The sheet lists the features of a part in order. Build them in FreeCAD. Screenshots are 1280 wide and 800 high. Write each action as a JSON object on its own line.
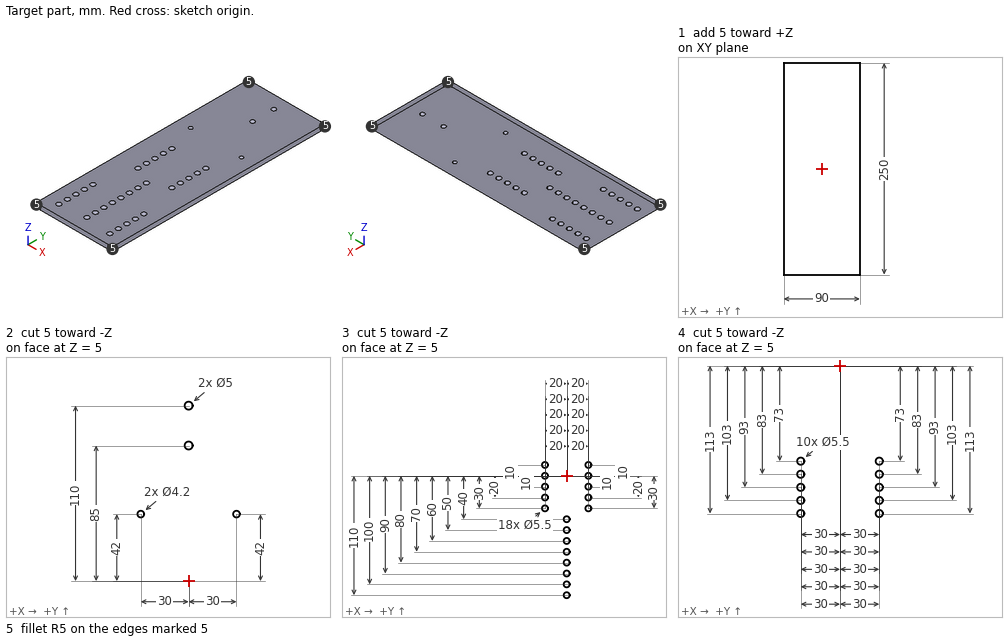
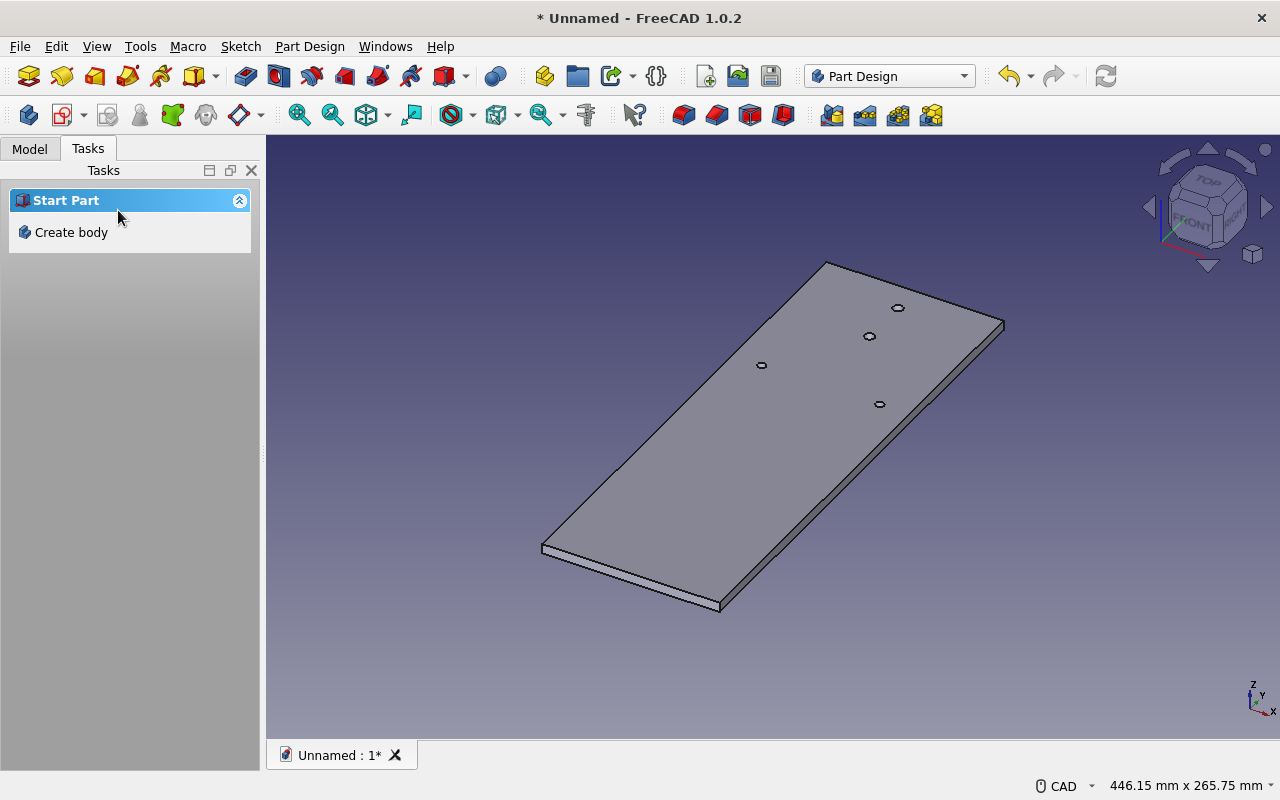
{"action": "left_click", "coordinate": [773, 431]}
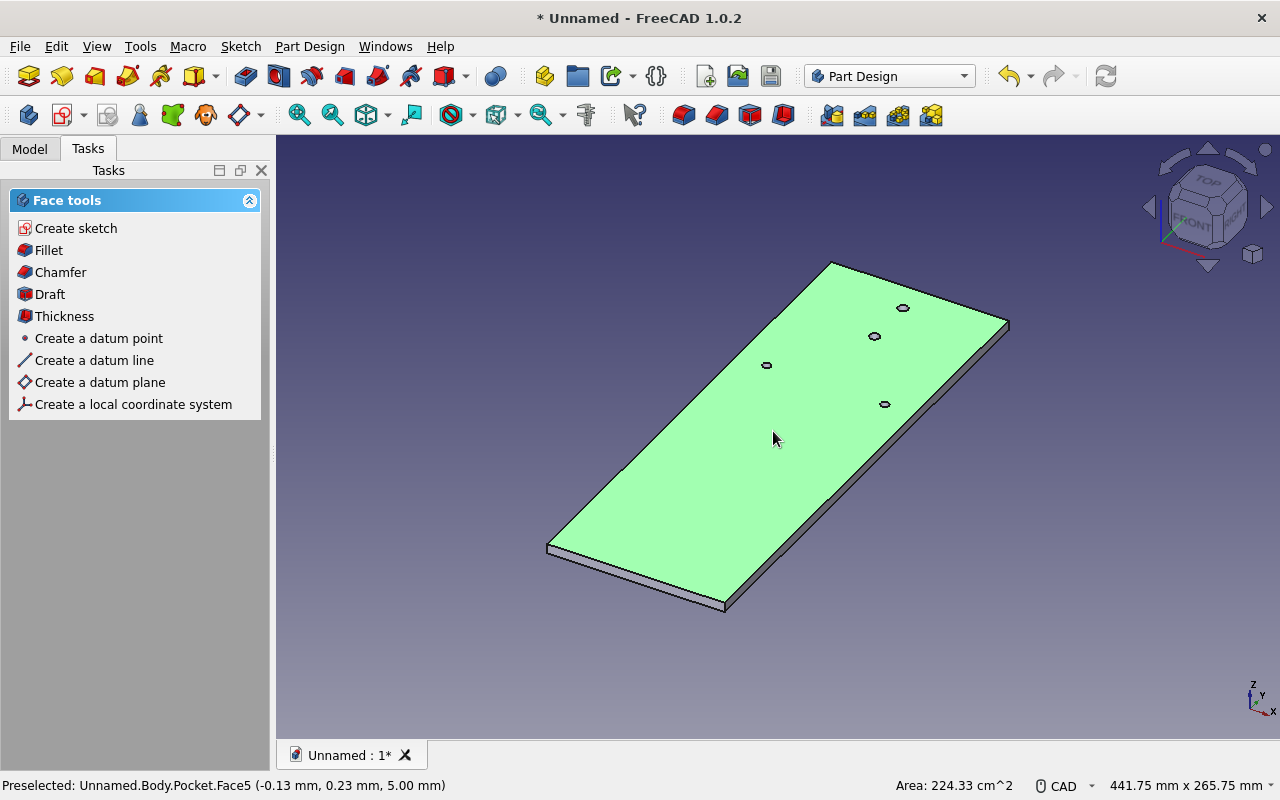
{"action": "left_click", "coordinate": [62, 116]}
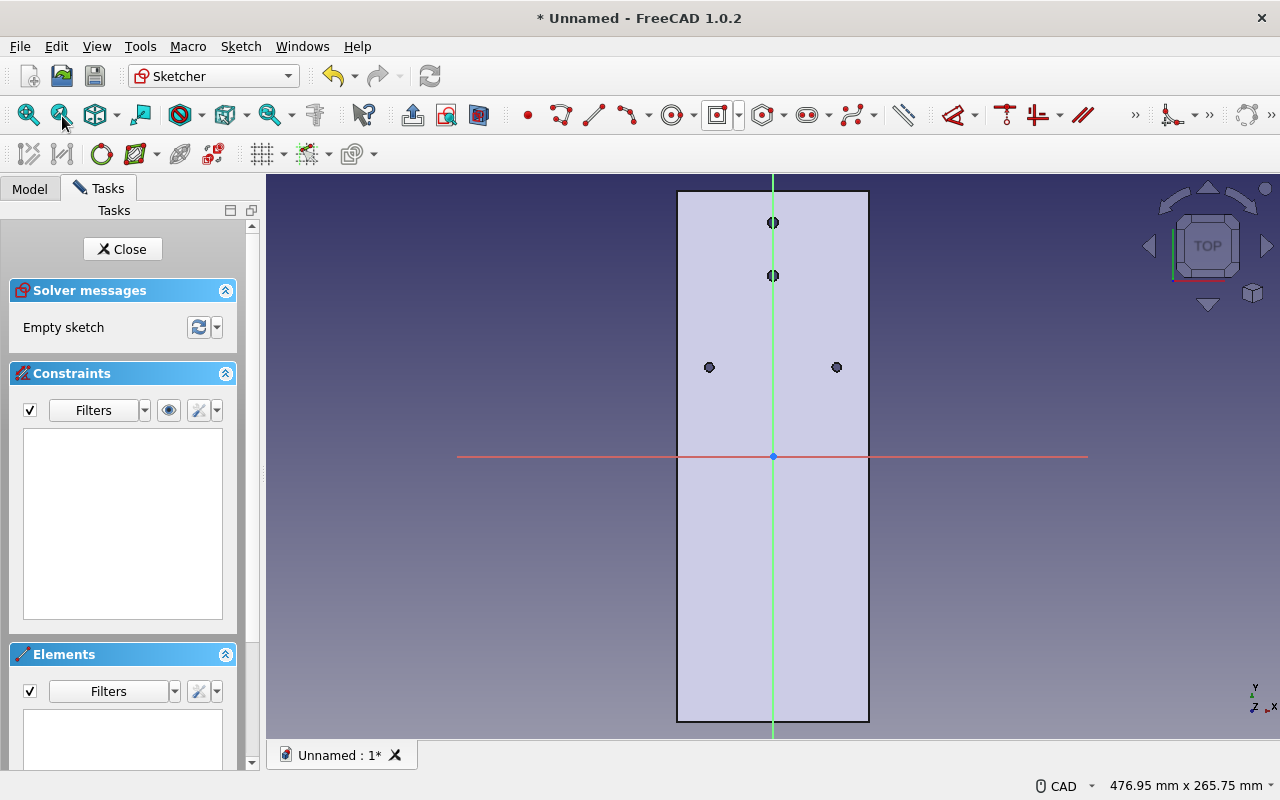
{"action": "scroll", "coordinate": [395, 202], "scroll_direction": "down", "scroll_amount": 1}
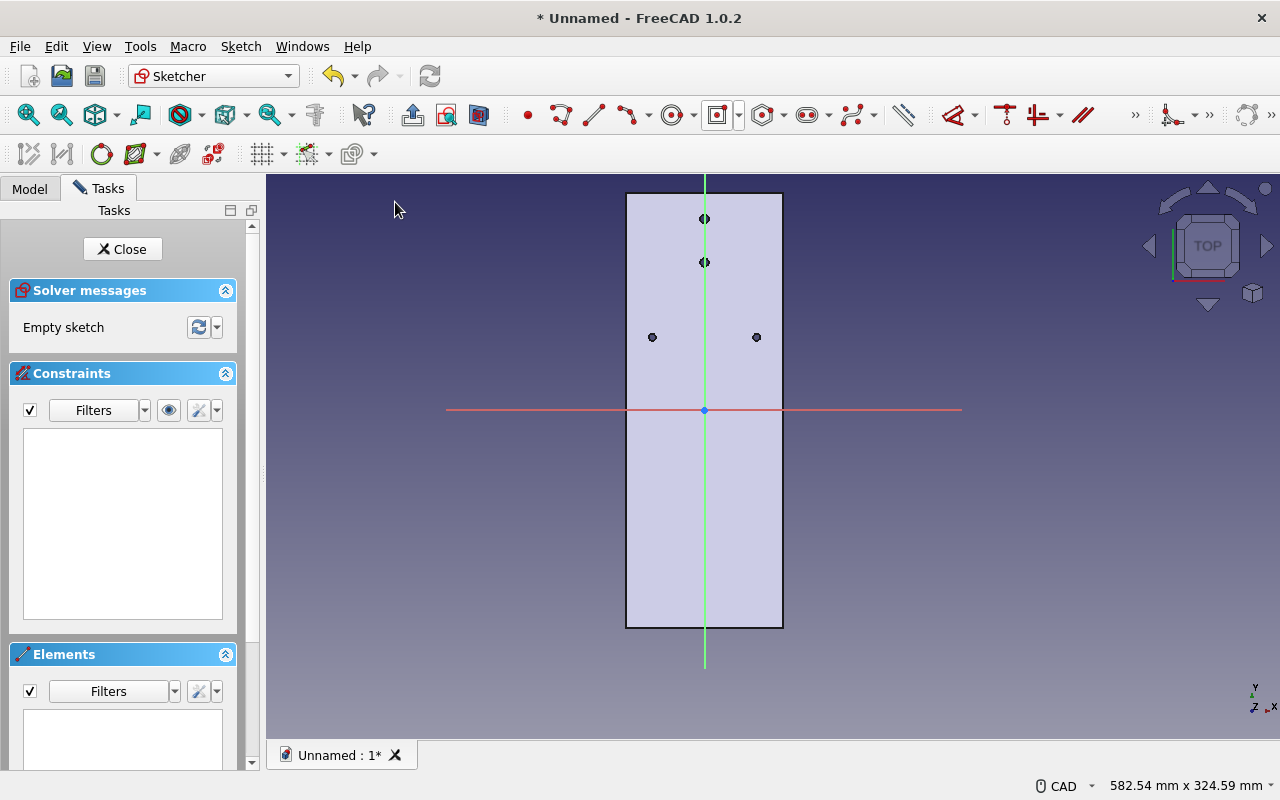
{"action": "scroll", "coordinate": [705, 581], "scroll_direction": "up", "scroll_amount": 2}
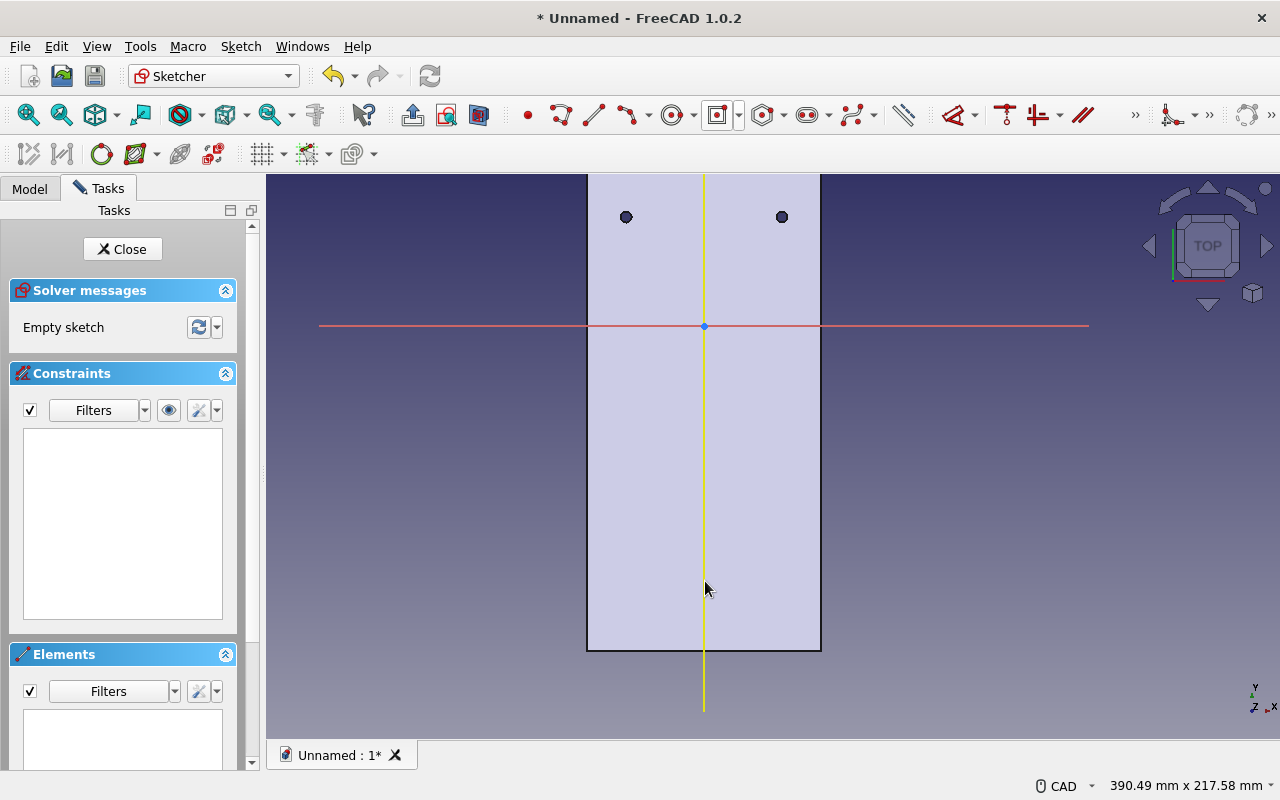
{"action": "key", "text": "g c"}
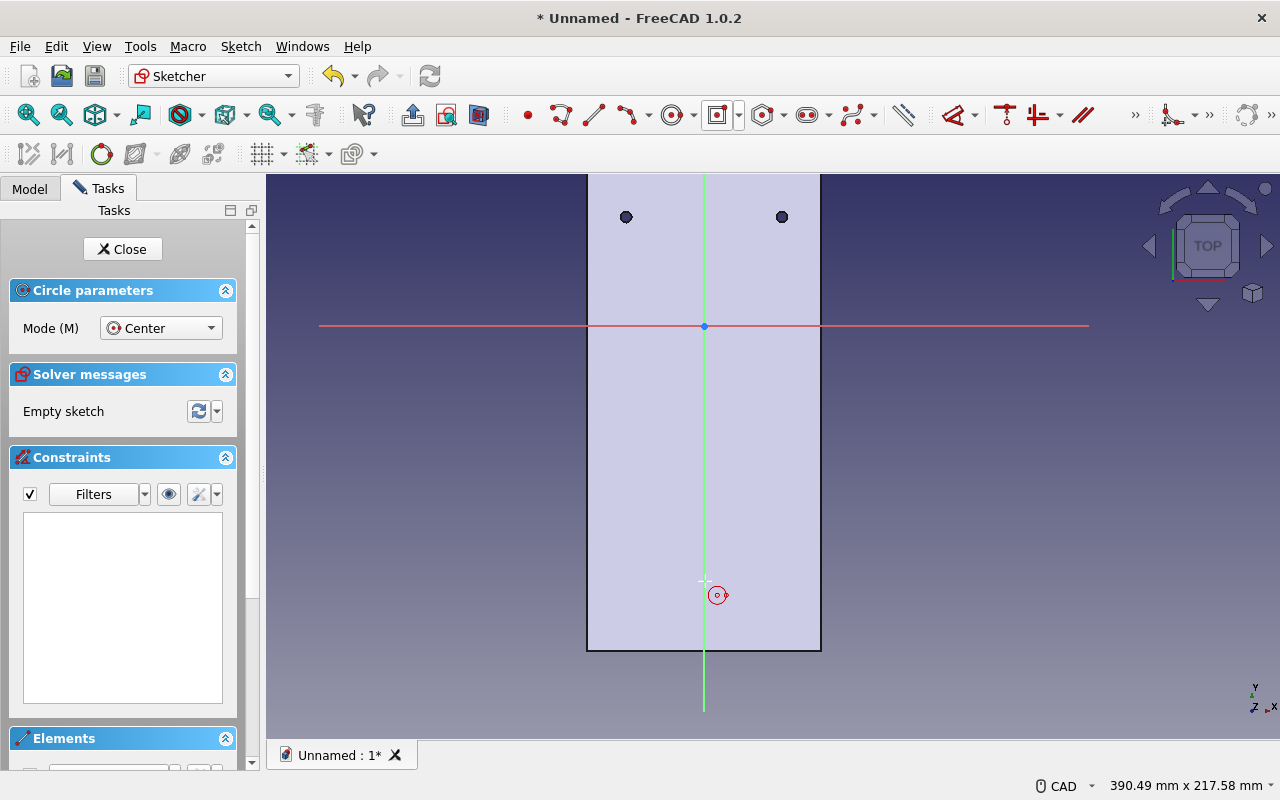
{"action": "scroll", "coordinate": [652, 404], "scroll_direction": "up", "scroll_amount": 6}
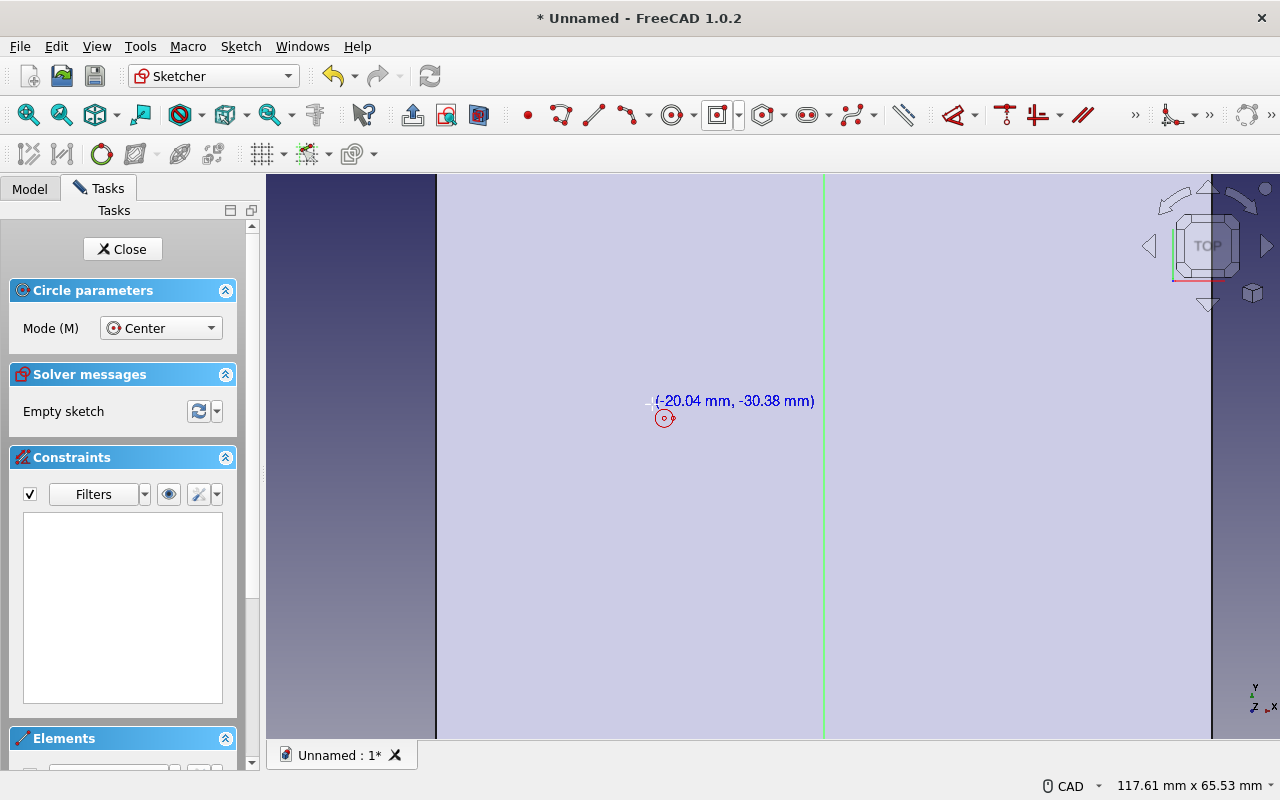
{"action": "left_click", "coordinate": [651, 403]}
{"action": "mouse_move", "coordinate": [668, 386]}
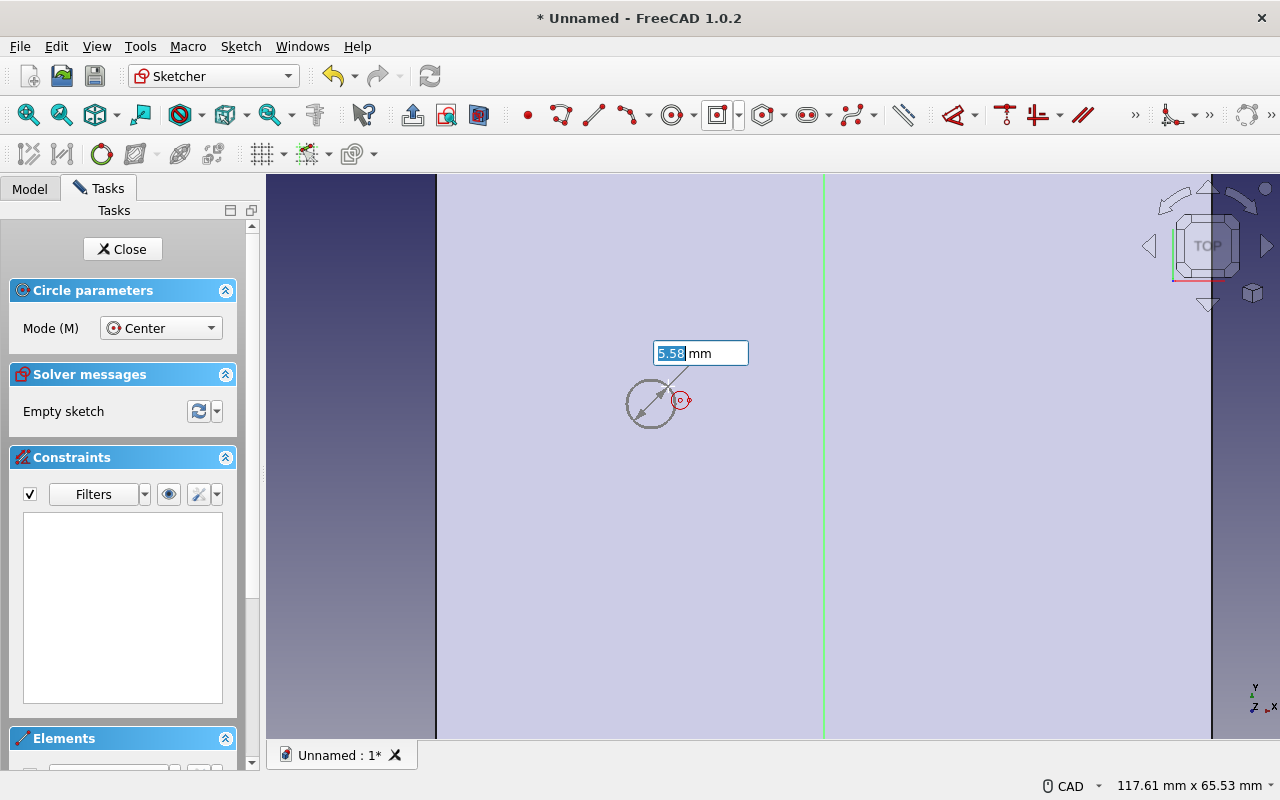
{"action": "type", "text": "5.5"}
{"action": "key", "text": "Return"}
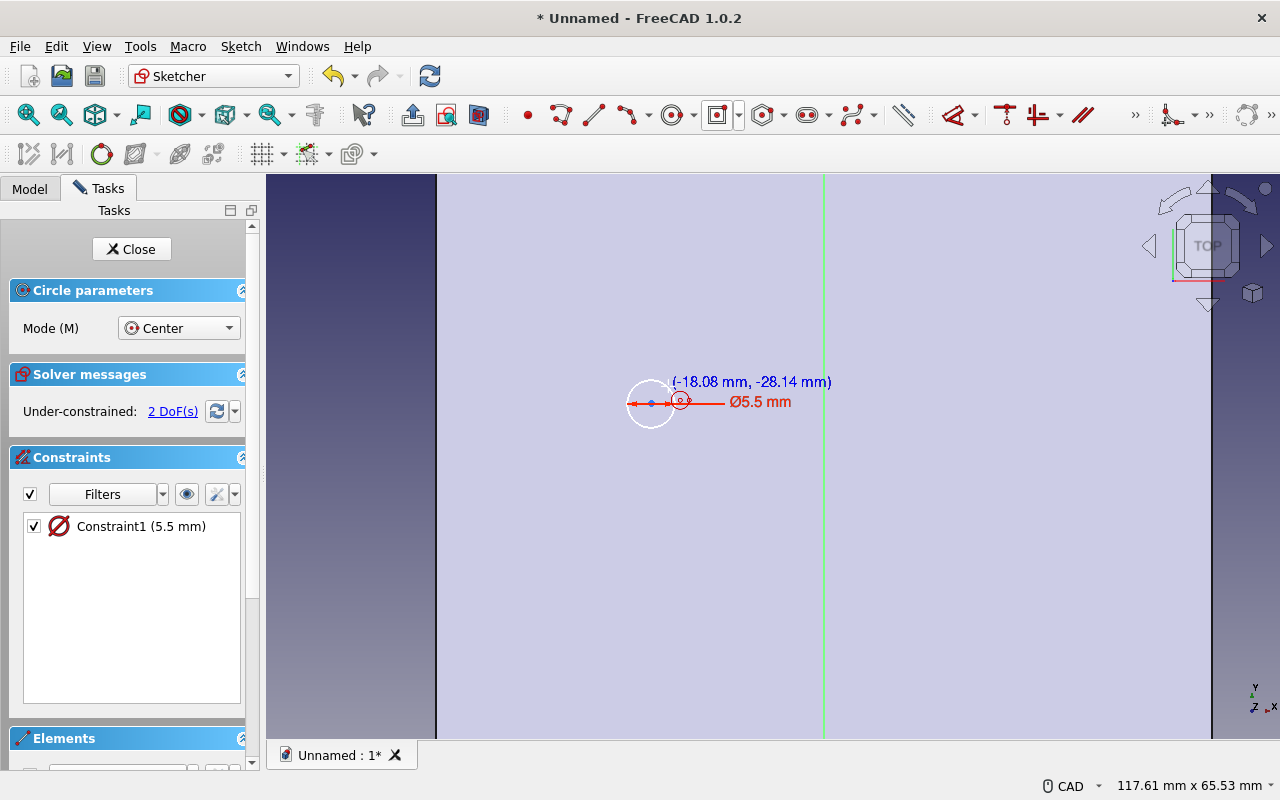
{"action": "left_click", "coordinate": [996, 403]}
{"action": "mouse_move", "coordinate": [1013, 386]}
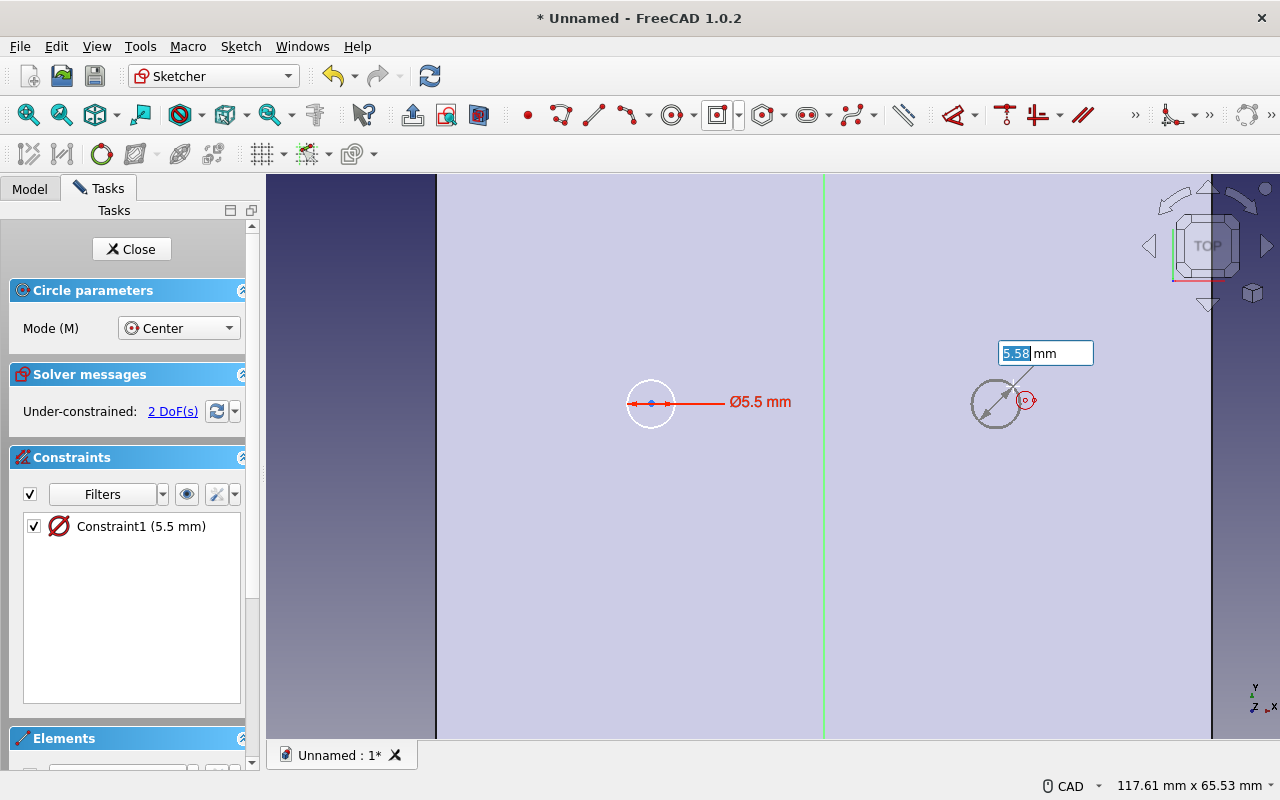
{"action": "type", "text": "5.5"}
{"action": "key", "text": "Return"}